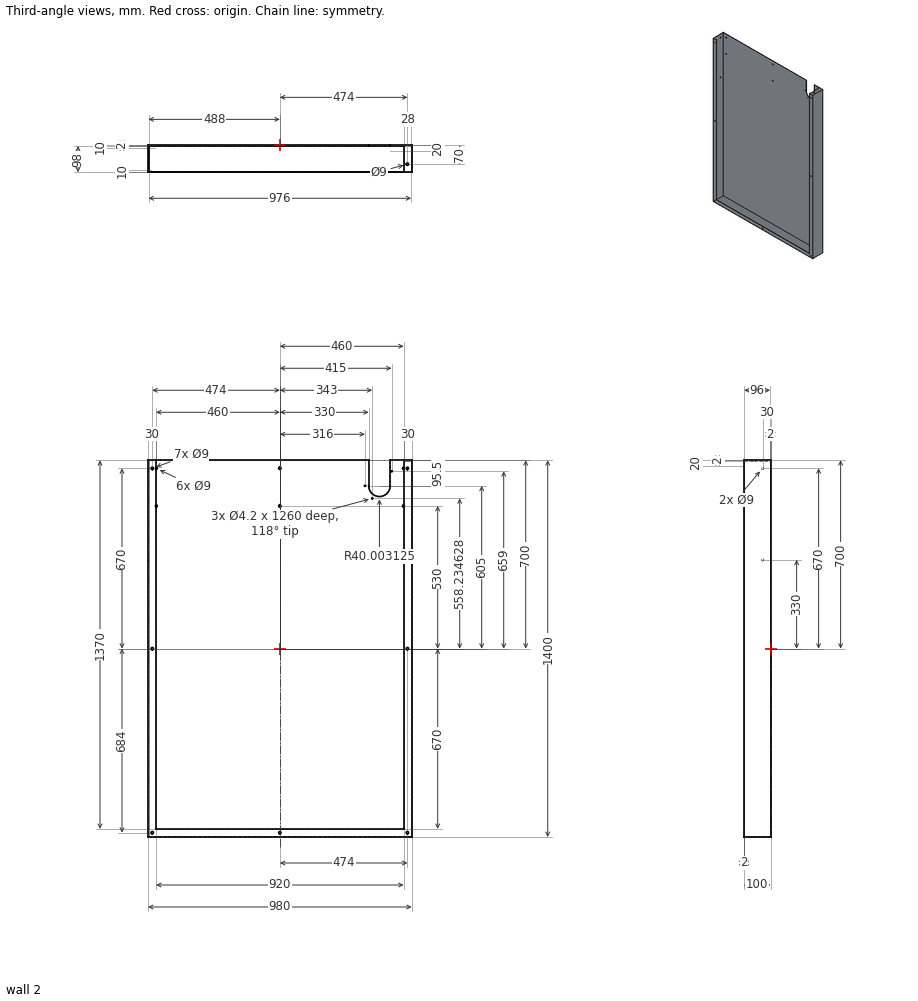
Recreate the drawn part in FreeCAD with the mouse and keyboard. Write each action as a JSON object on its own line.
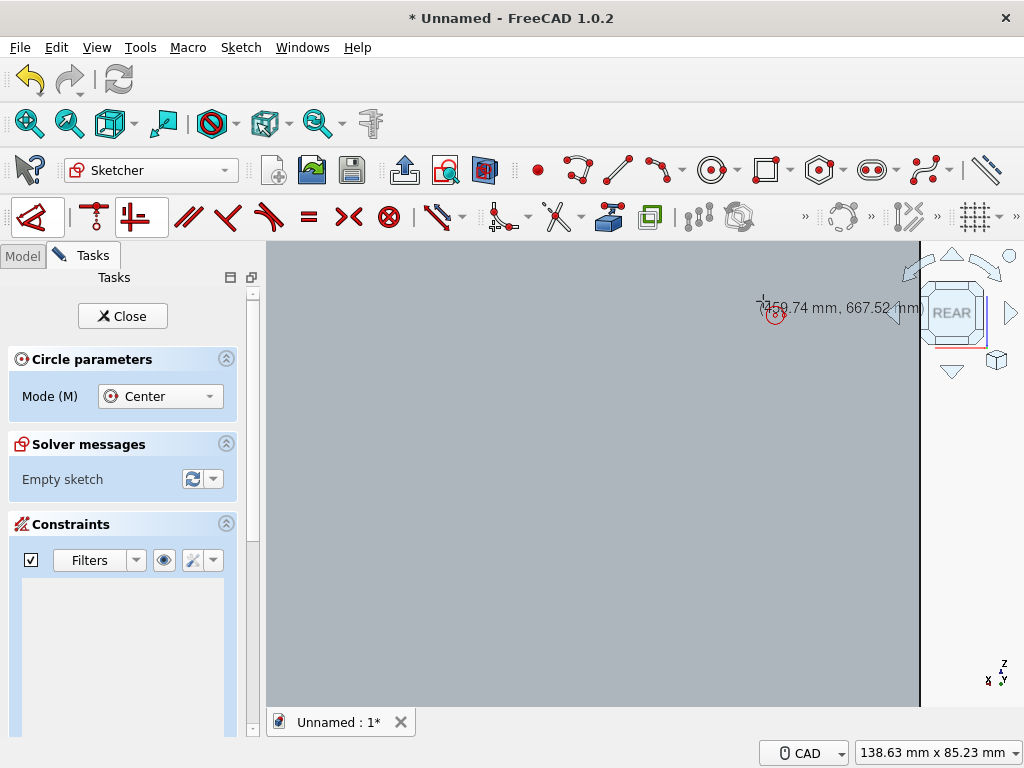
{"action": "scroll", "coordinate": [764, 342], "scroll_direction": "down", "scroll_amount": 13}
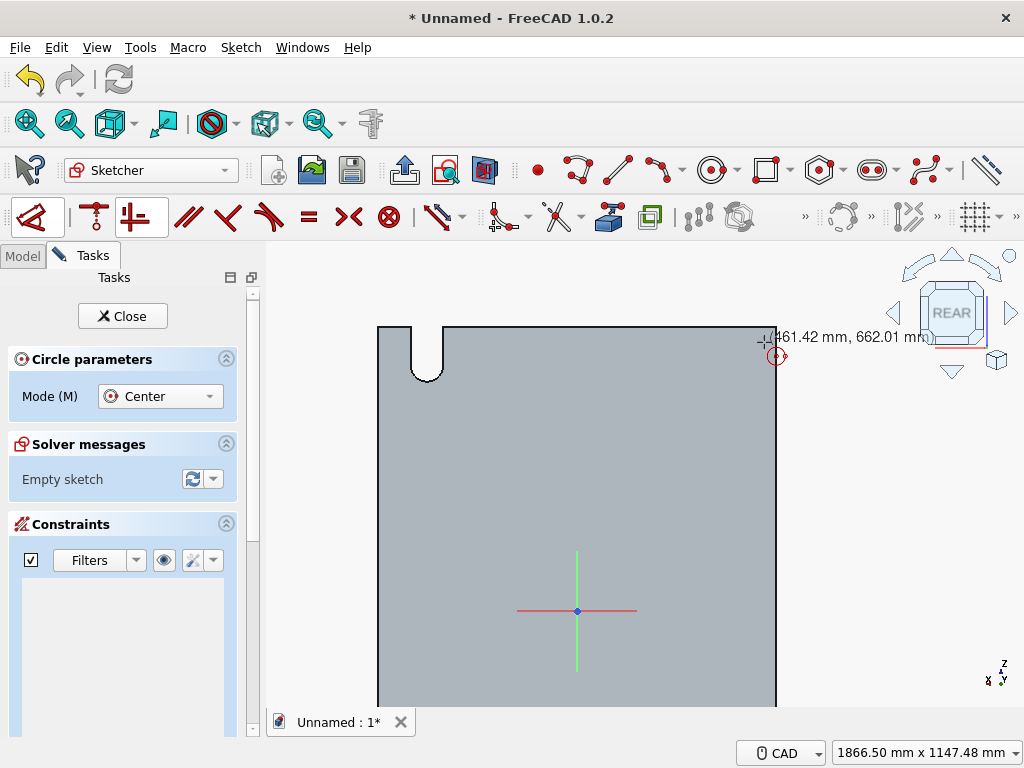
{"action": "left_click", "coordinate": [764, 339]}
{"action": "mouse_move", "coordinate": [765, 338]}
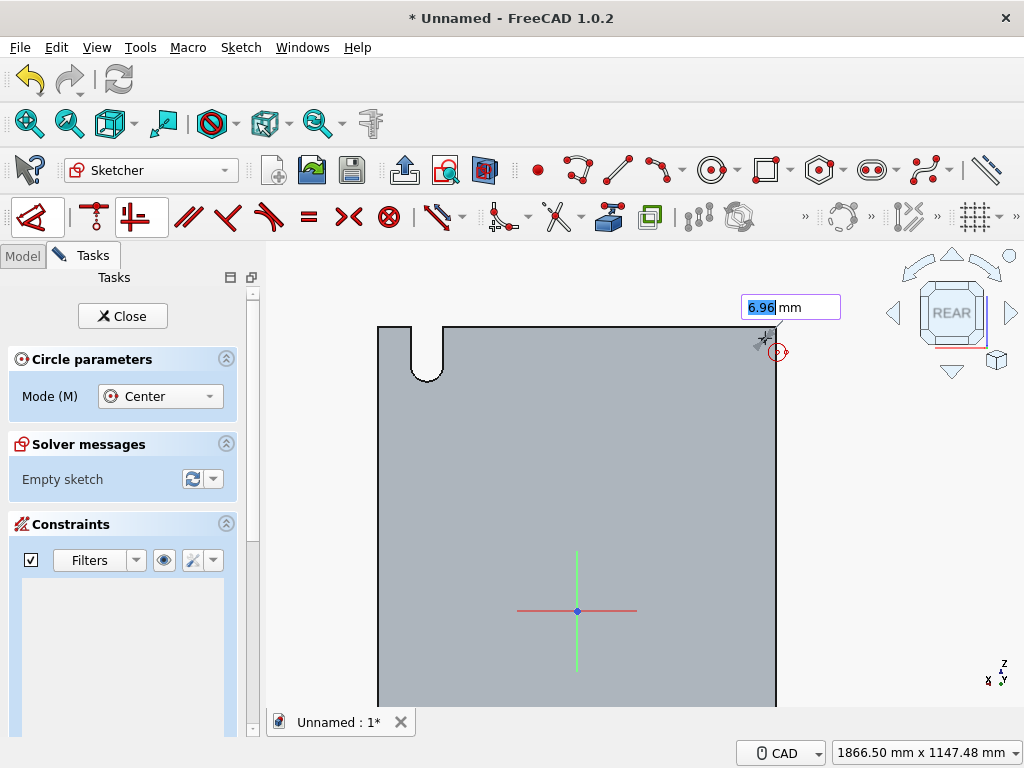
{"action": "type", "text": "9"}
{"action": "key", "text": "Return"}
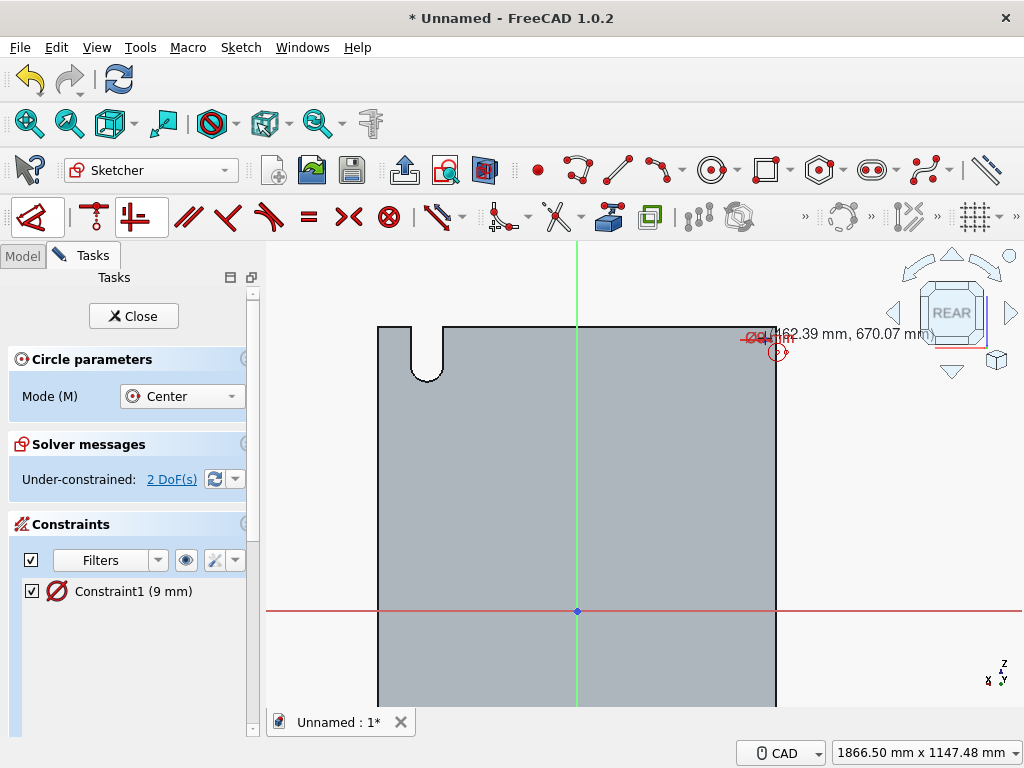
{"action": "scroll", "coordinate": [577, 396], "scroll_direction": "up", "scroll_amount": 13}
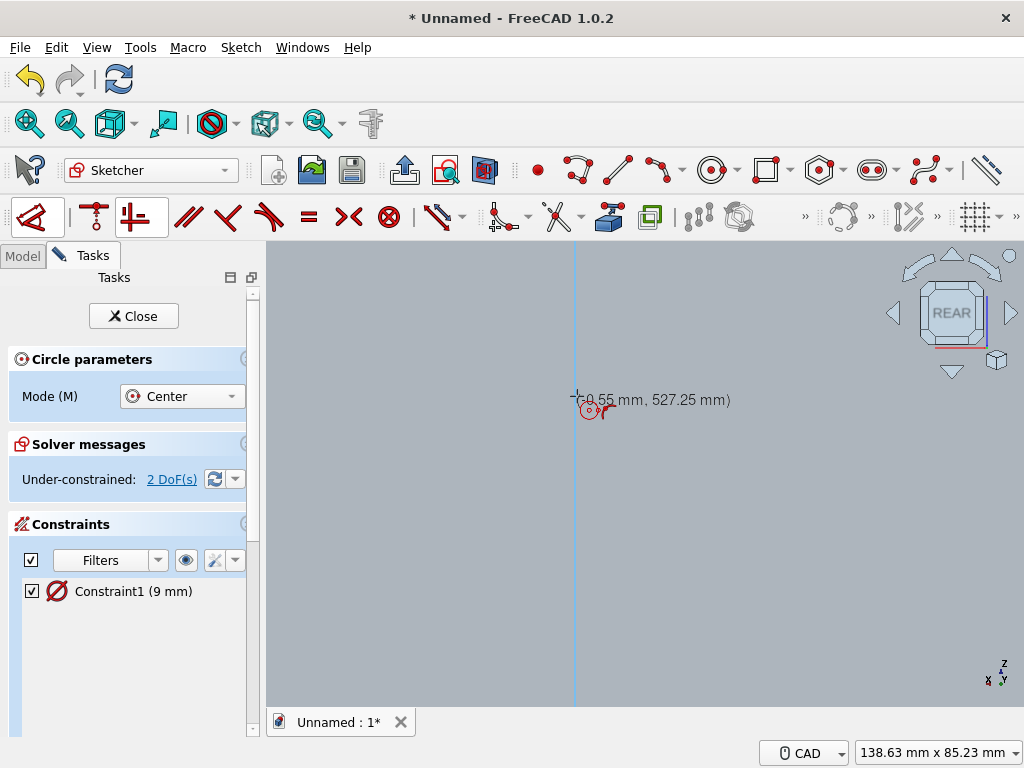
{"action": "scroll", "coordinate": [577, 396], "scroll_direction": "down", "scroll_amount": 13}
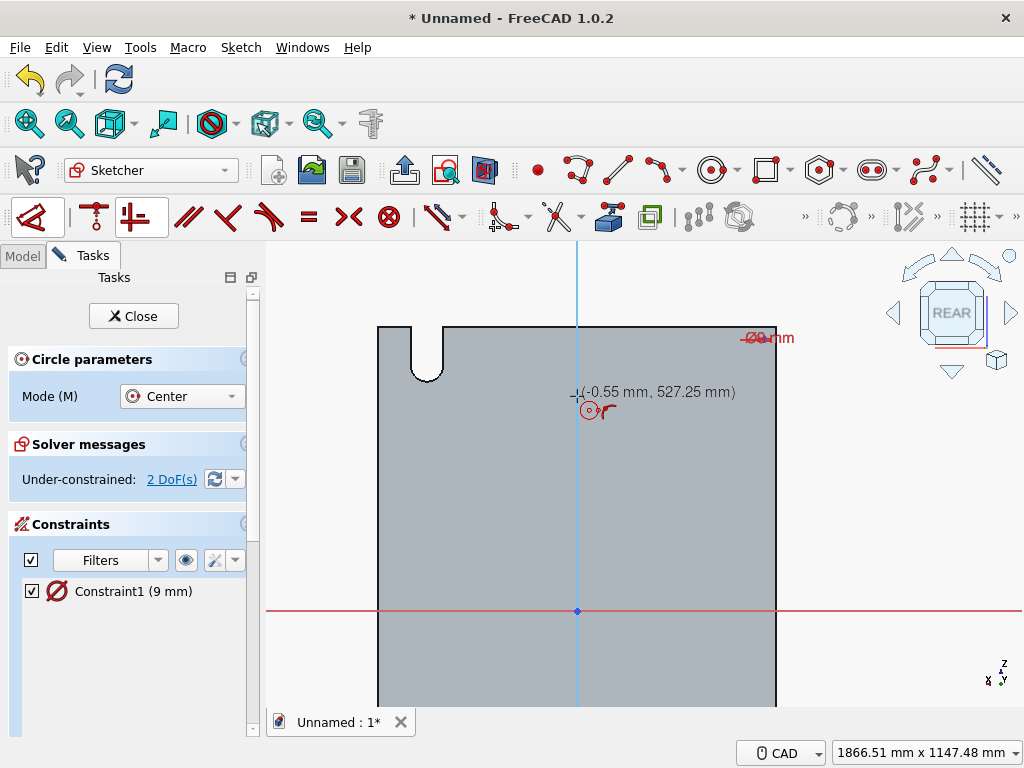
{"action": "left_click", "coordinate": [577, 396]}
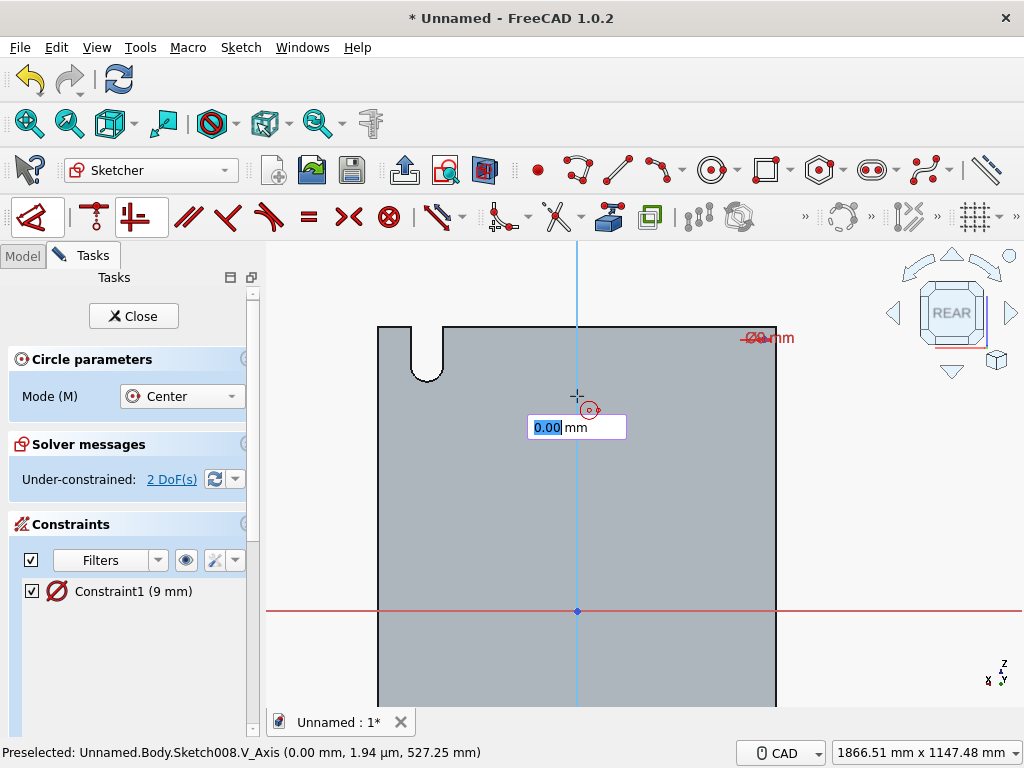
{"action": "scroll", "coordinate": [579, 395], "scroll_direction": "up", "scroll_amount": 12}
{"action": "mouse_move", "coordinate": [574, 395]}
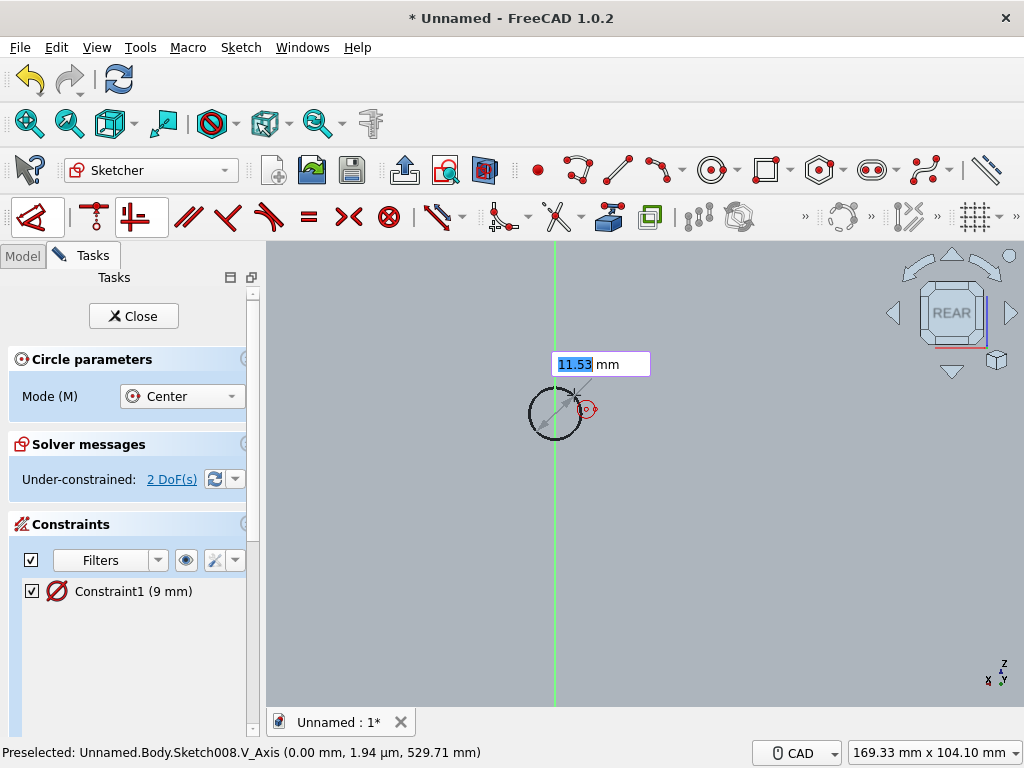
{"action": "type", "text": "9"}
{"action": "key", "text": "Return"}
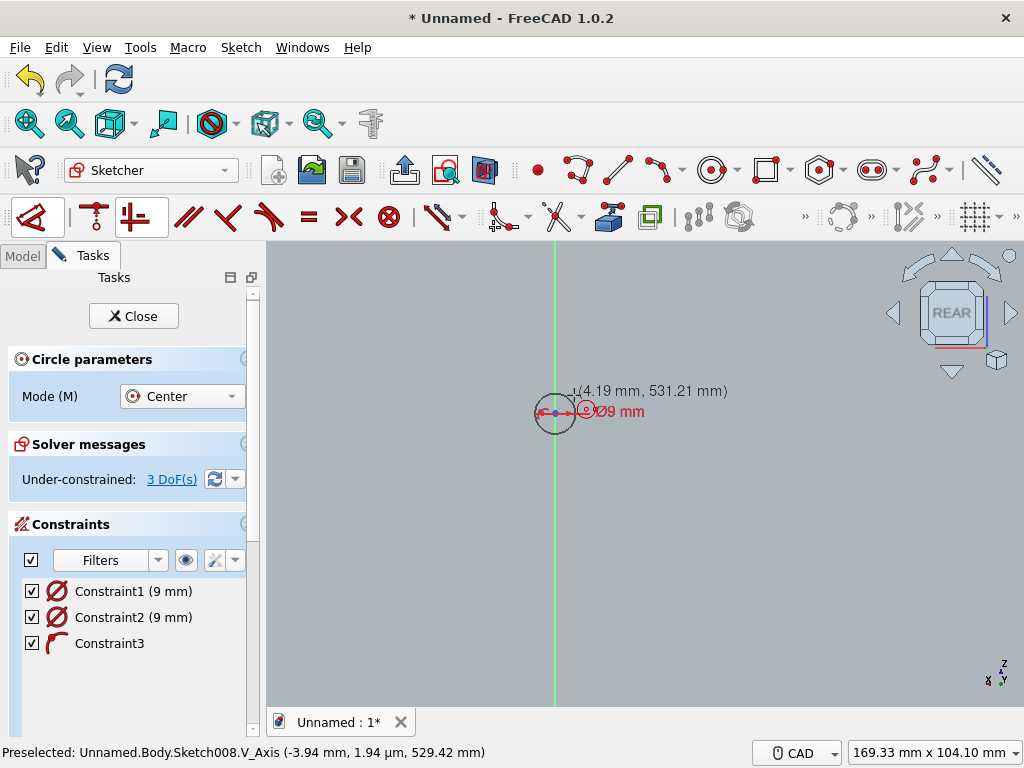
{"action": "scroll", "coordinate": [579, 395], "scroll_direction": "down", "scroll_amount": 12}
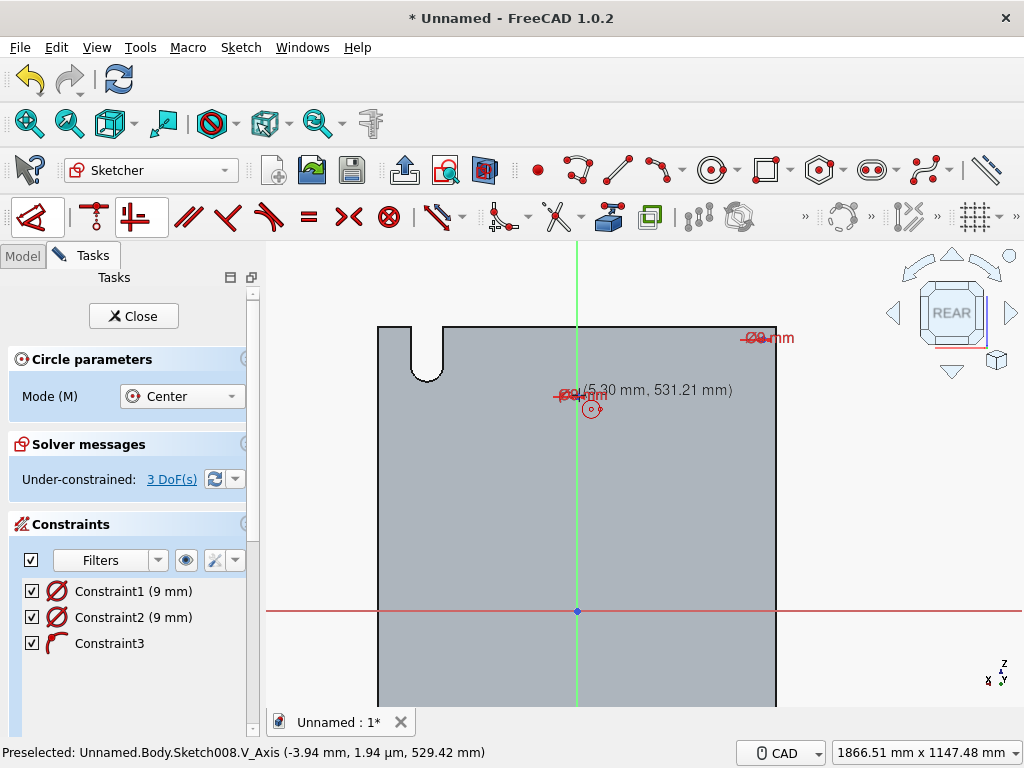
{"action": "scroll", "coordinate": [390, 396], "scroll_direction": "up", "scroll_amount": 13}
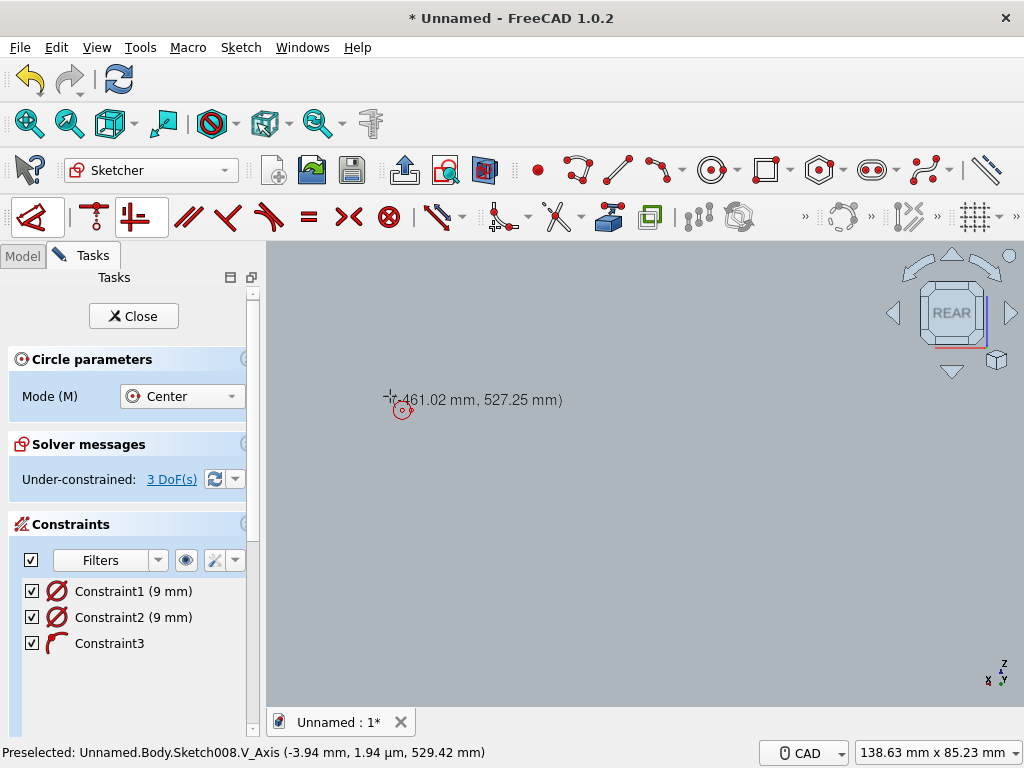
{"action": "scroll", "coordinate": [389, 396], "scroll_direction": "down", "scroll_amount": 13}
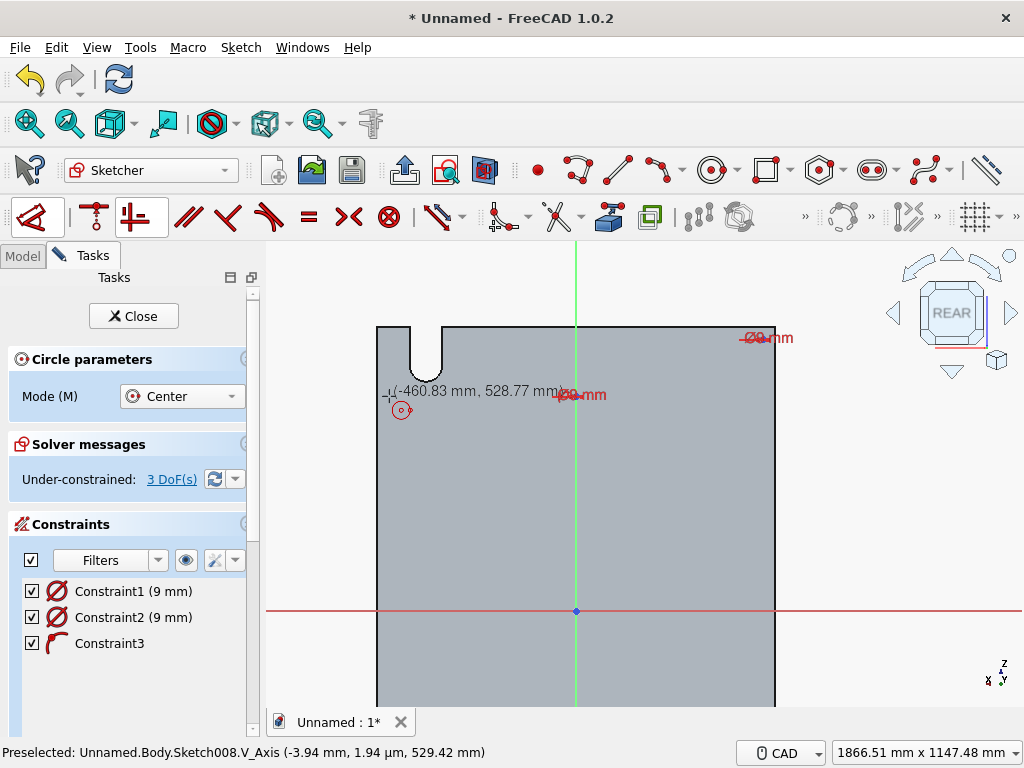
{"action": "left_click", "coordinate": [389, 396]}
{"action": "mouse_move", "coordinate": [391, 395]}